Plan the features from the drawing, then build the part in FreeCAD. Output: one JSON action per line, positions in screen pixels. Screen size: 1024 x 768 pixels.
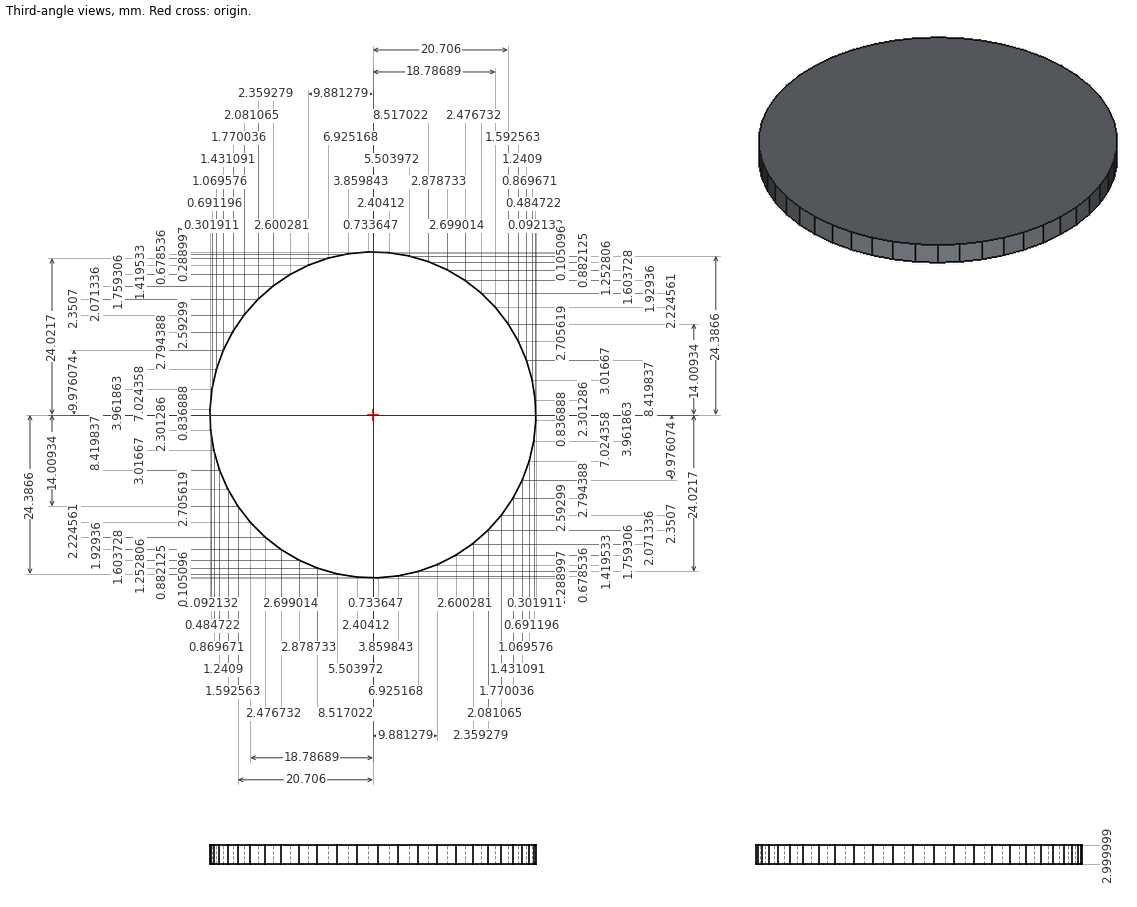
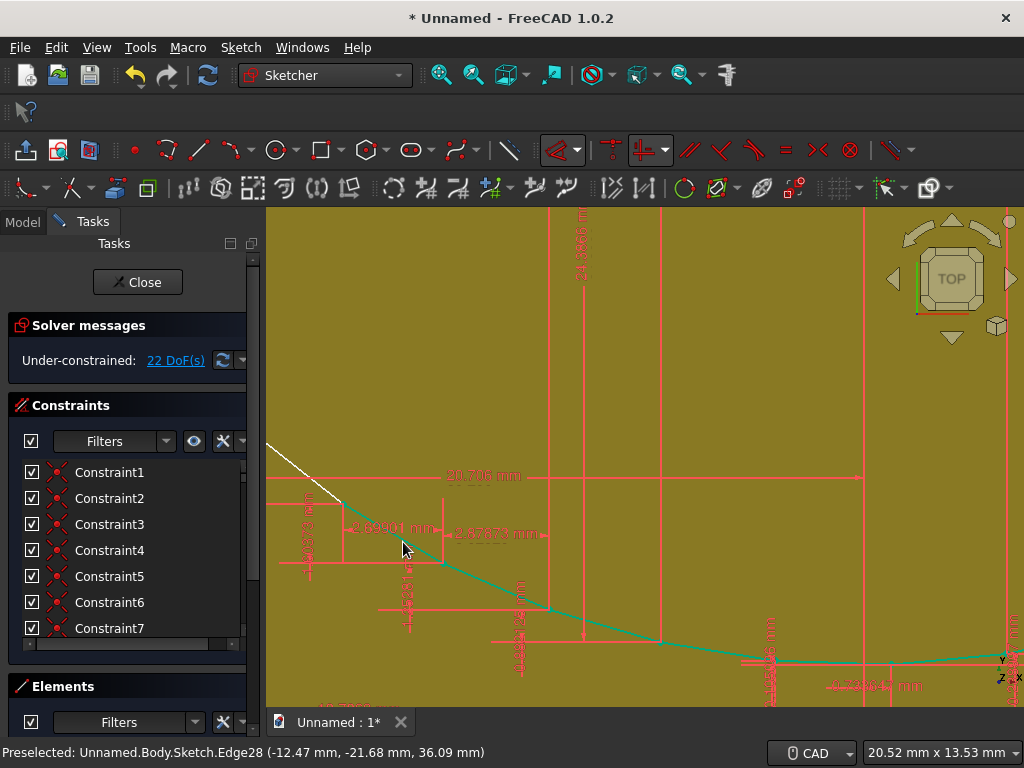
{"action": "left_click", "coordinate": [316, 483]}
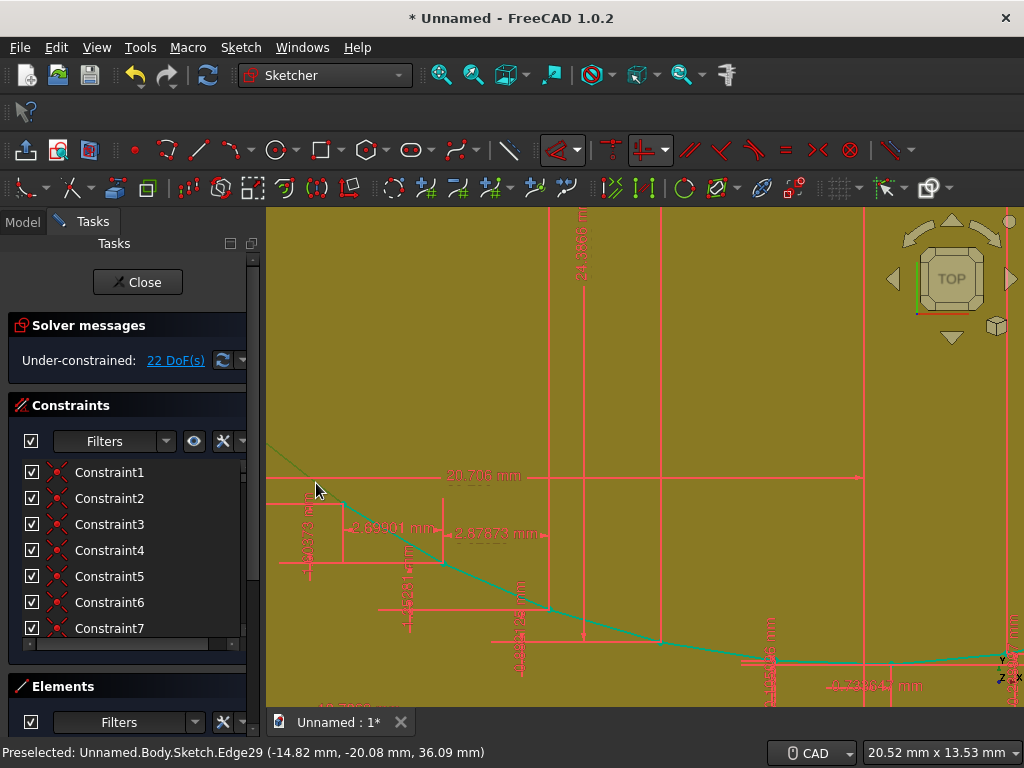
{"action": "left_click", "coordinate": [580, 150]}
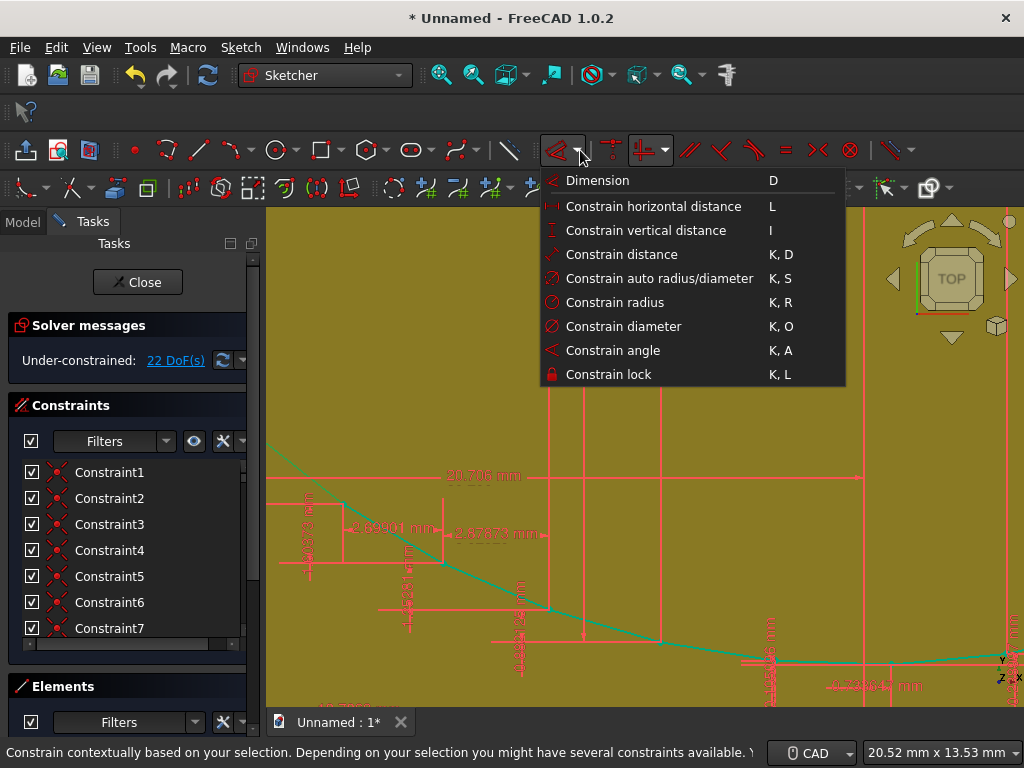
{"action": "left_click", "coordinate": [693, 206]}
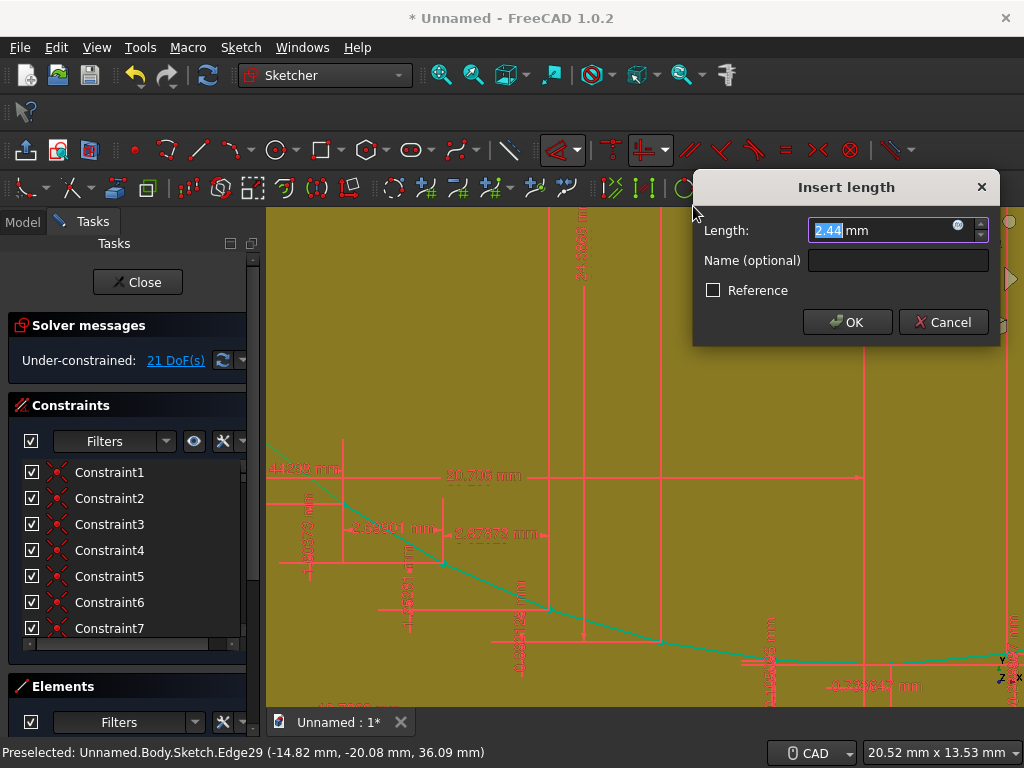
{"action": "type", "text": "2.476732"}
{"action": "key", "text": "Return"}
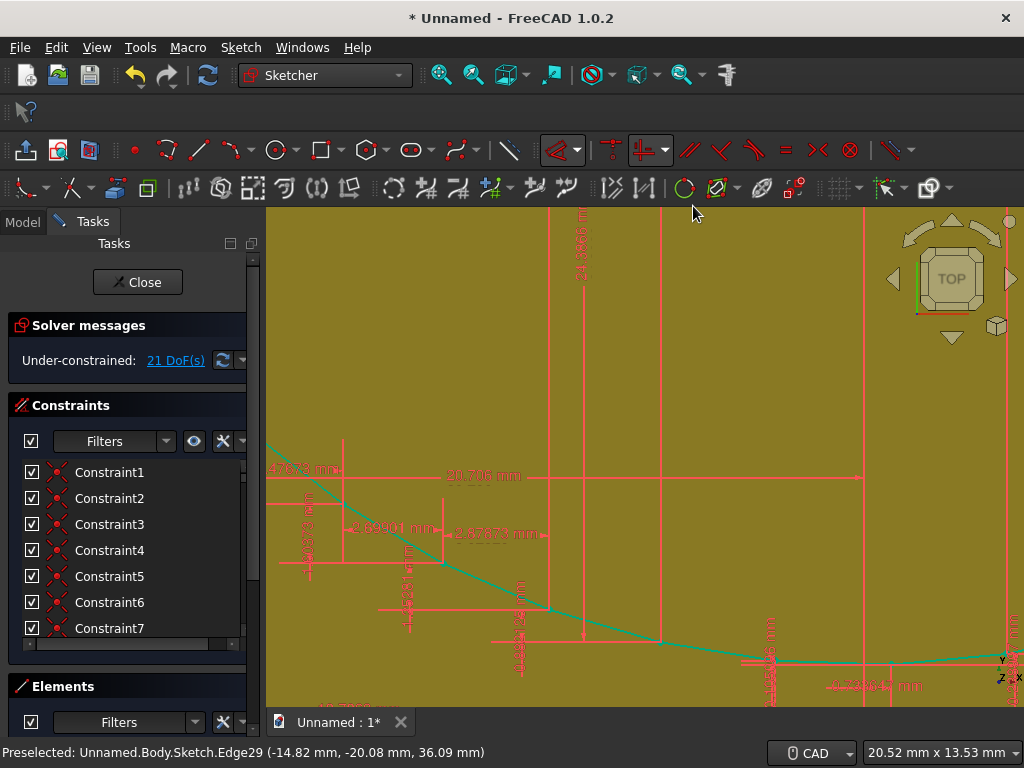
{"action": "scroll", "coordinate": [520, 599], "scroll_direction": "down", "scroll_amount": 9}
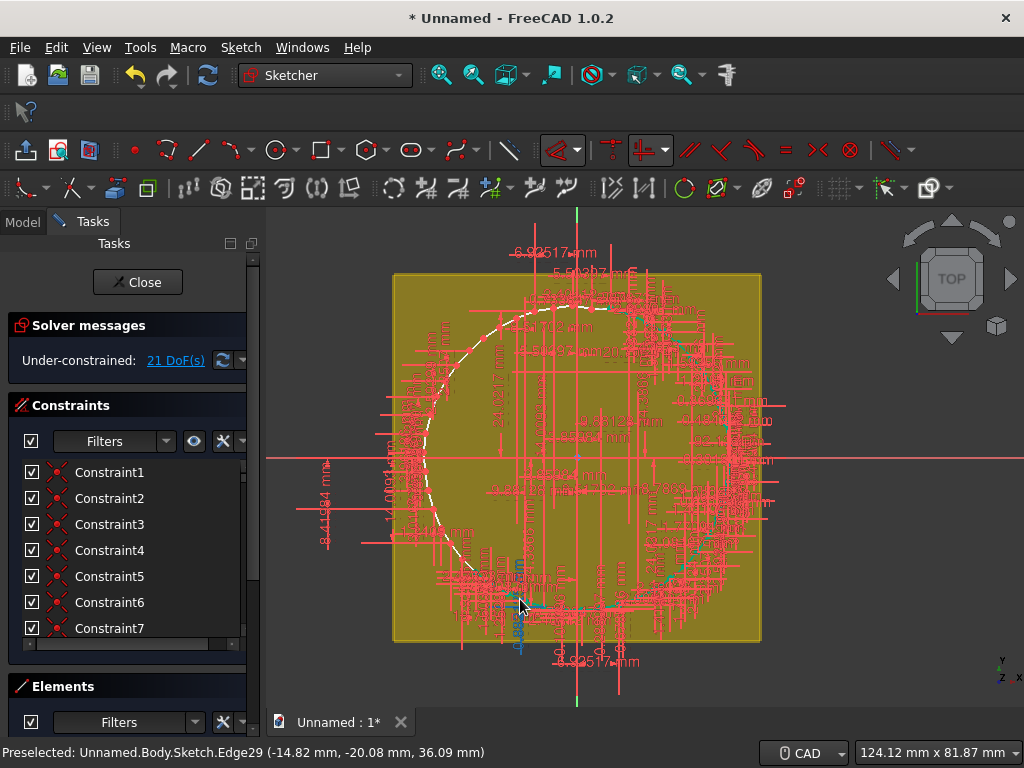
{"action": "scroll", "coordinate": [472, 568], "scroll_direction": "up", "scroll_amount": 6}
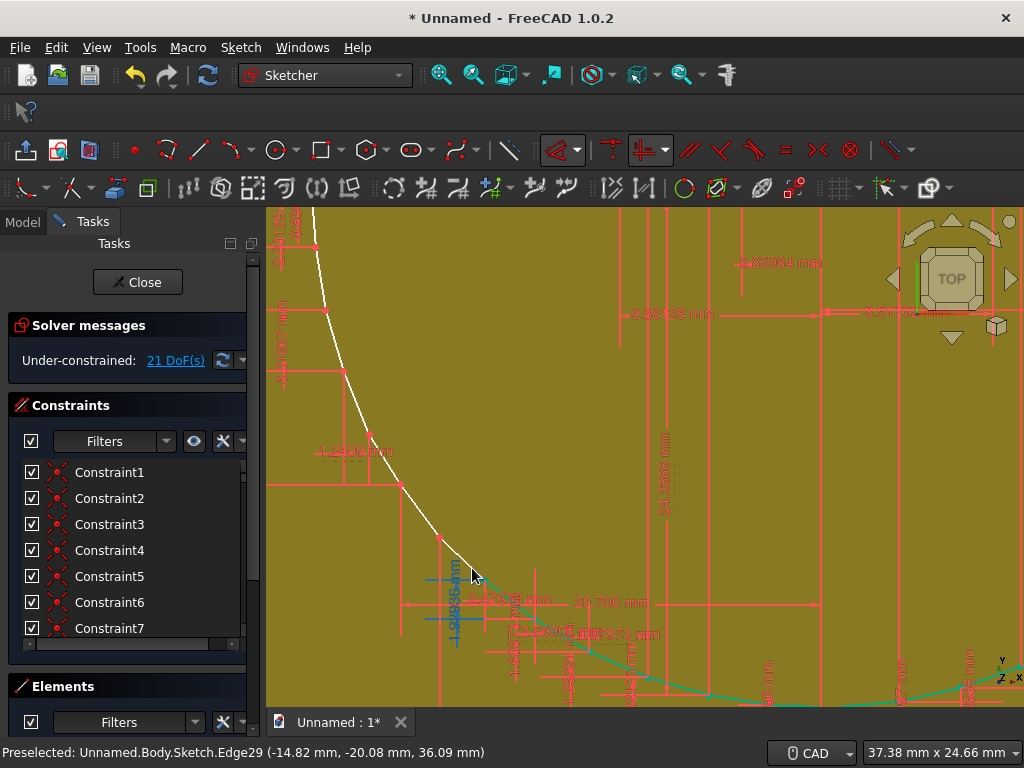
{"action": "left_click", "coordinate": [471, 567]}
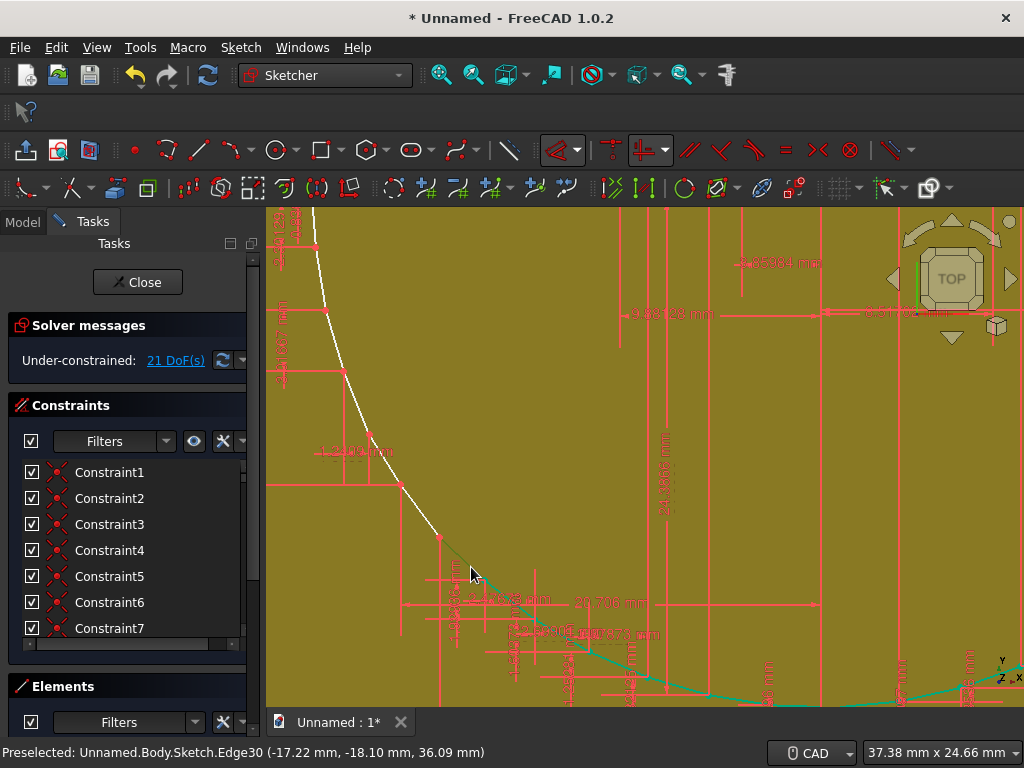
{"action": "key", "text": "i"}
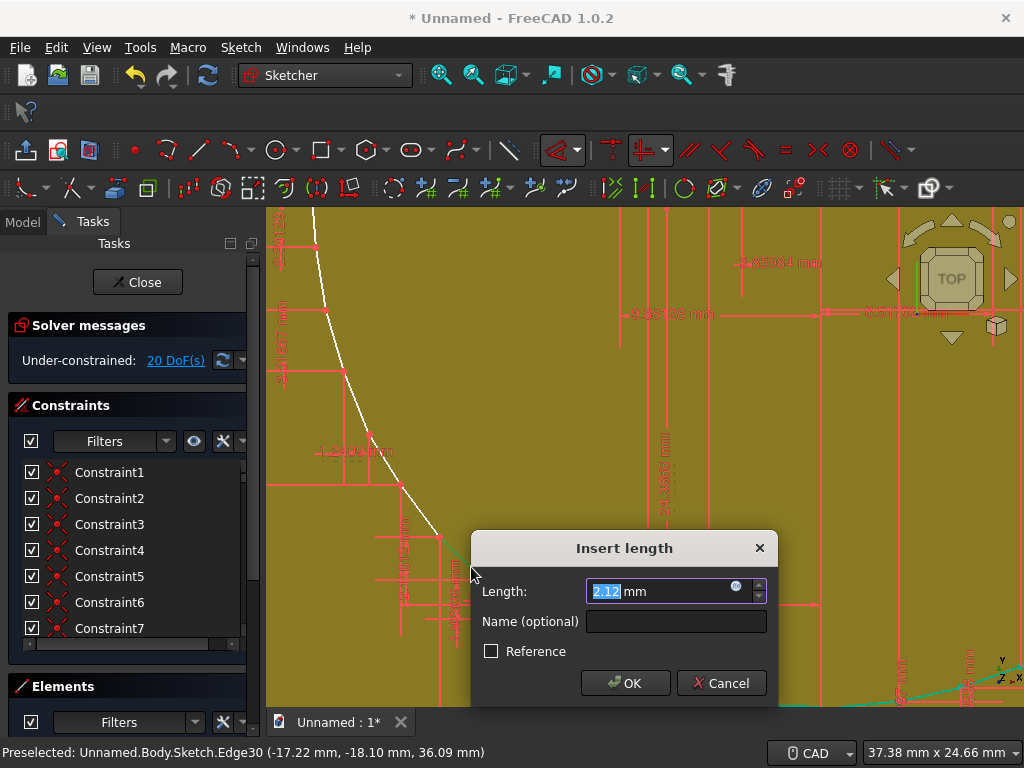
{"action": "type", "text": "2.224561"}
{"action": "key", "text": "Return"}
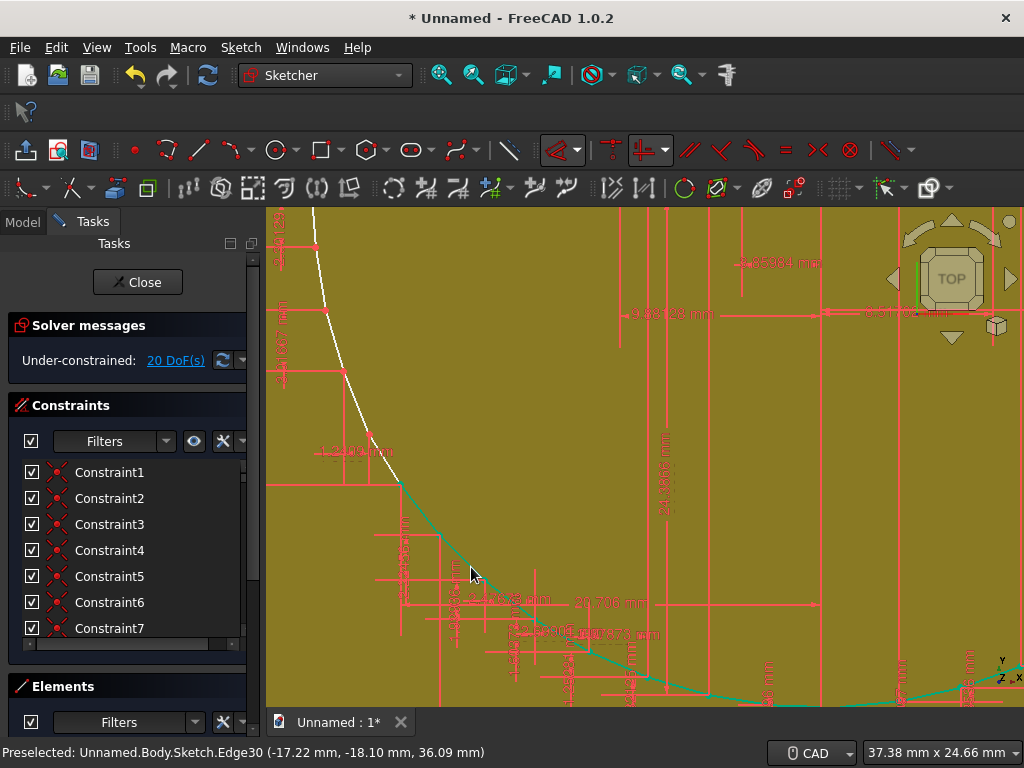
{"action": "scroll", "coordinate": [391, 470], "scroll_direction": "up", "scroll_amount": 2}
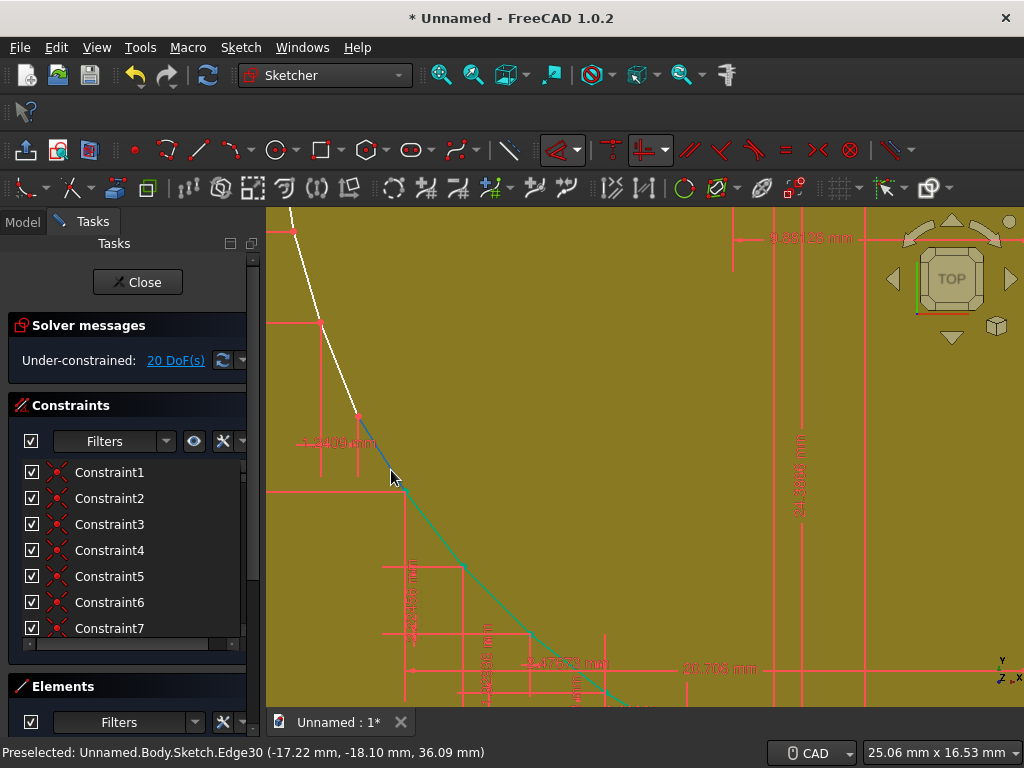
{"action": "left_click", "coordinate": [391, 469]}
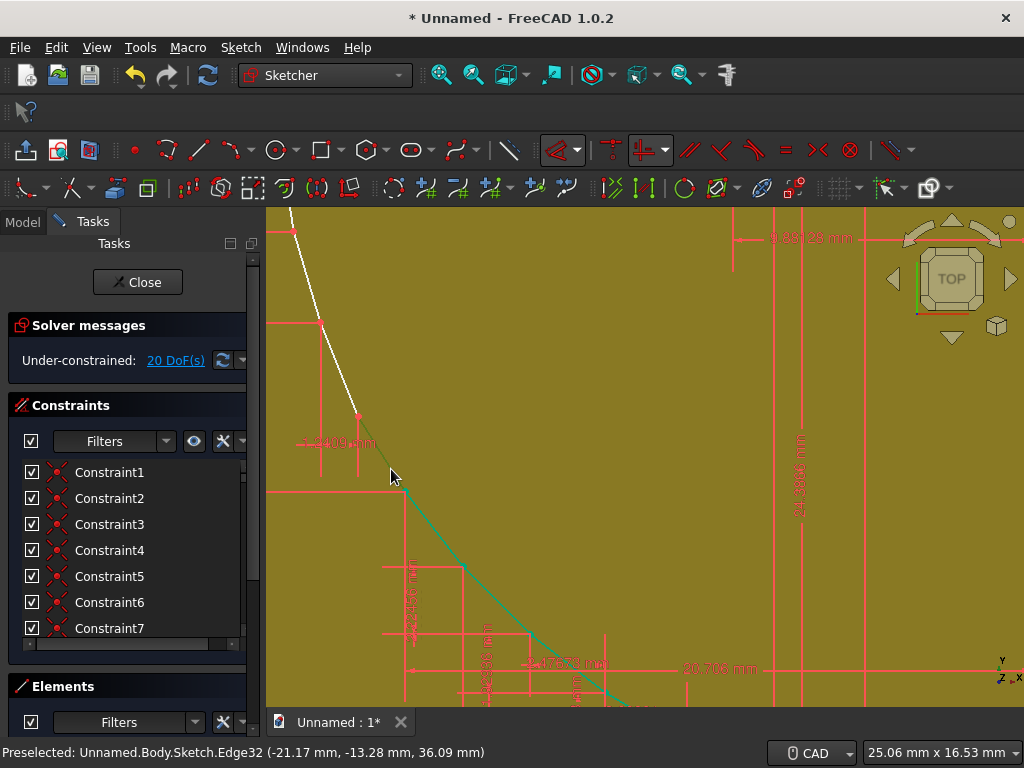
{"action": "left_click", "coordinate": [580, 150]}